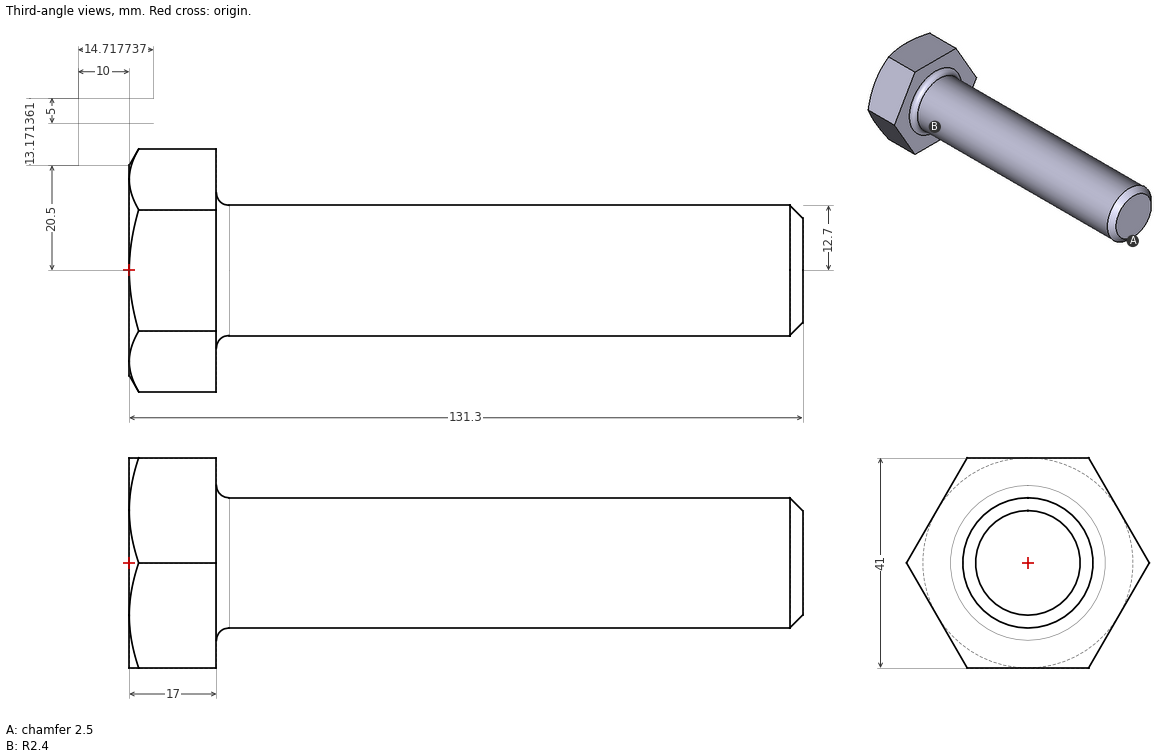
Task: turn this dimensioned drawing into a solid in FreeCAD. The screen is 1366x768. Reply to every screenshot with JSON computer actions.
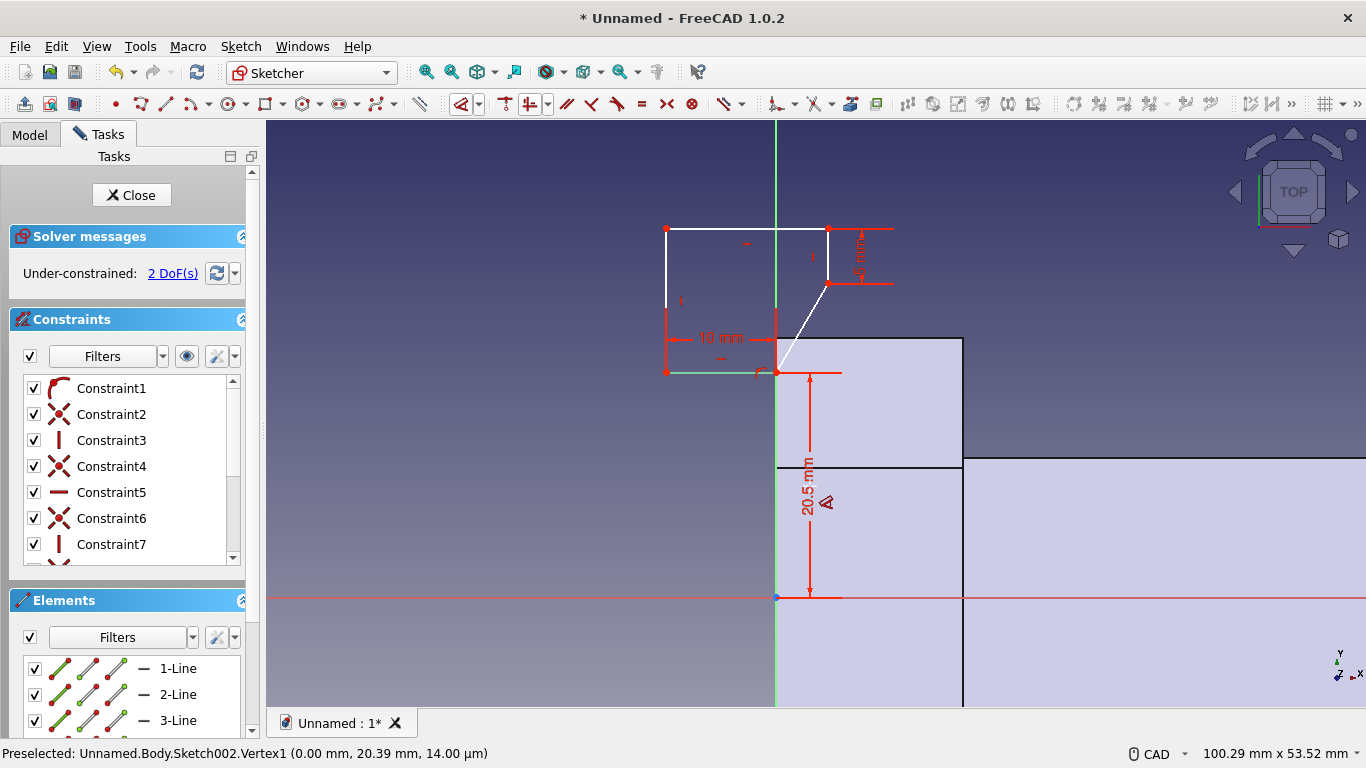
{"action": "left_click", "coordinate": [780, 229]}
{"action": "left_click", "coordinate": [747, 195]}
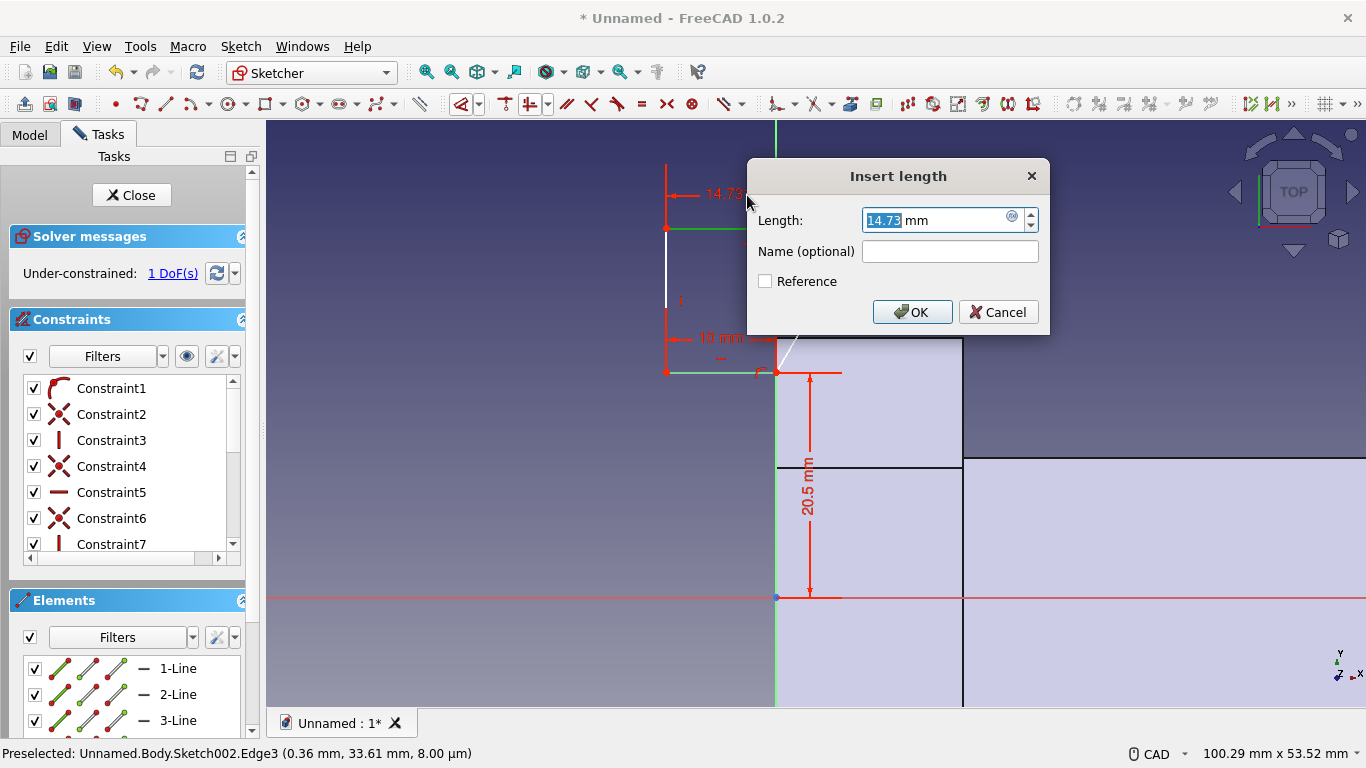
{"action": "type", "text": "14.717737"}
{"action": "key", "text": "Return"}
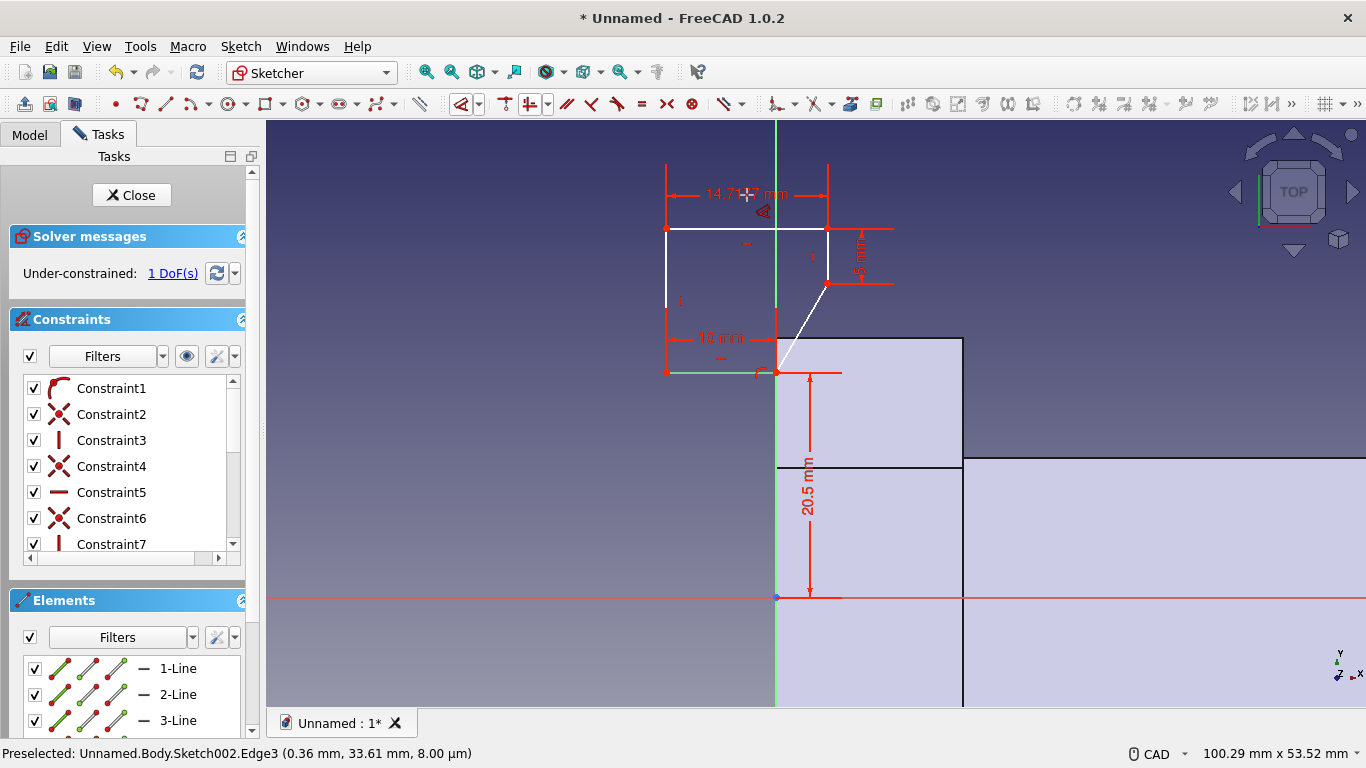
{"action": "left_click", "coordinate": [666, 272]}
{"action": "left_click", "coordinate": [632, 301]}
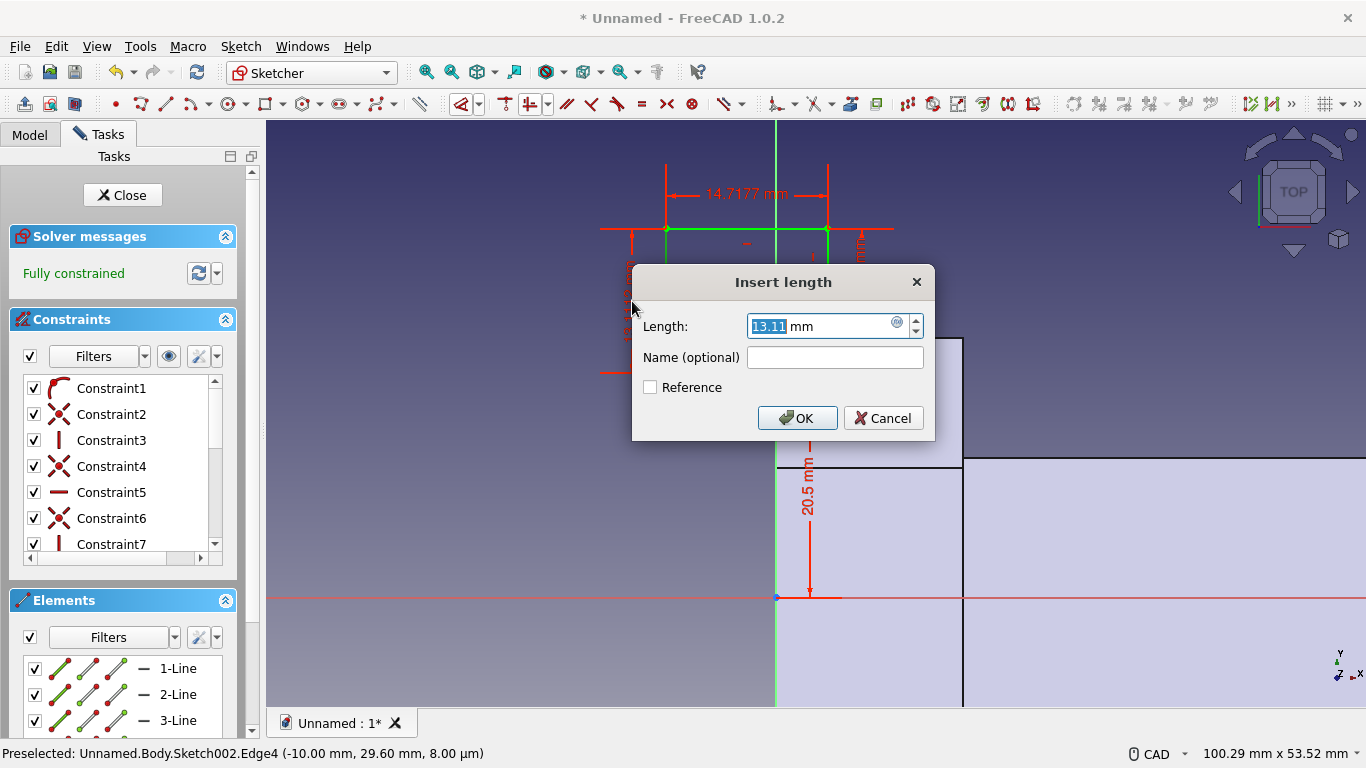
{"action": "type", "text": "13.171361"}
{"action": "key", "text": "Return"}
{"action": "key", "text": "Escape"}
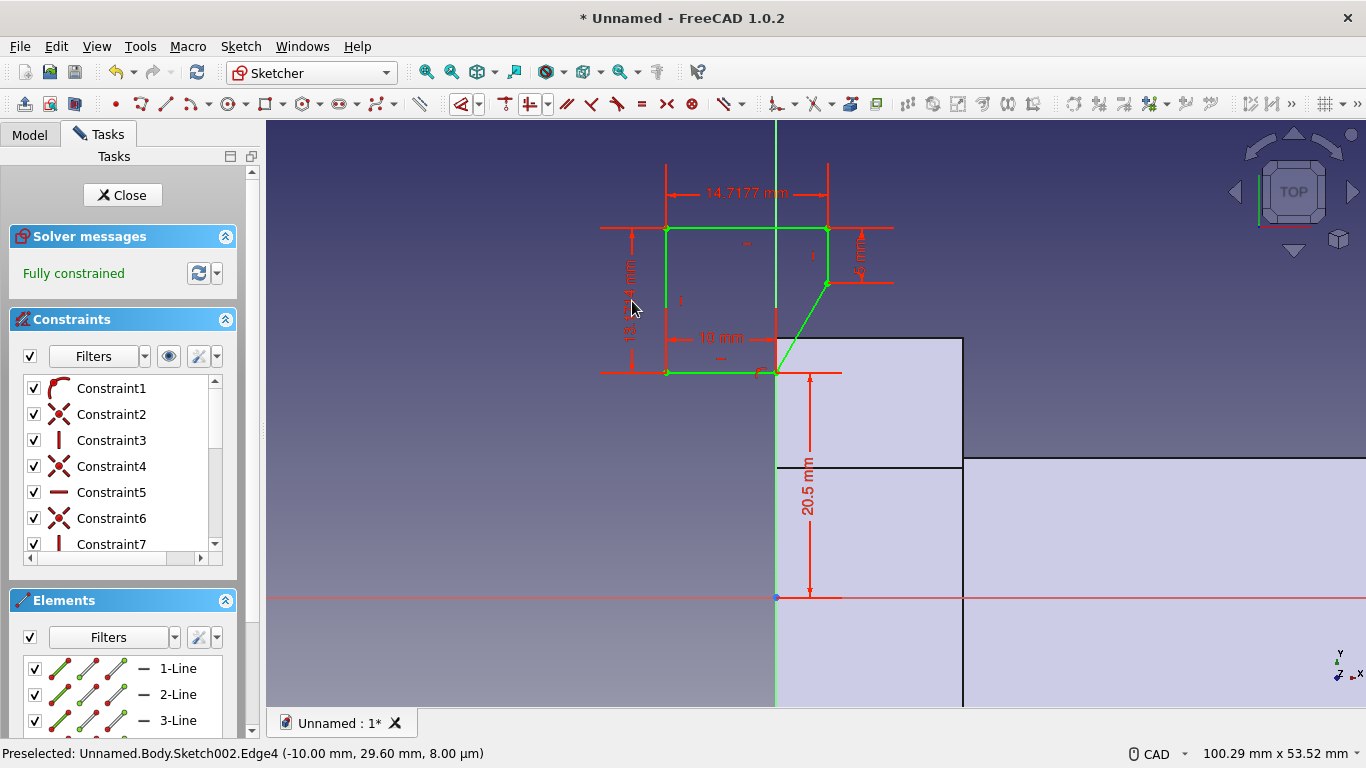
{"action": "left_click", "coordinate": [123, 195]}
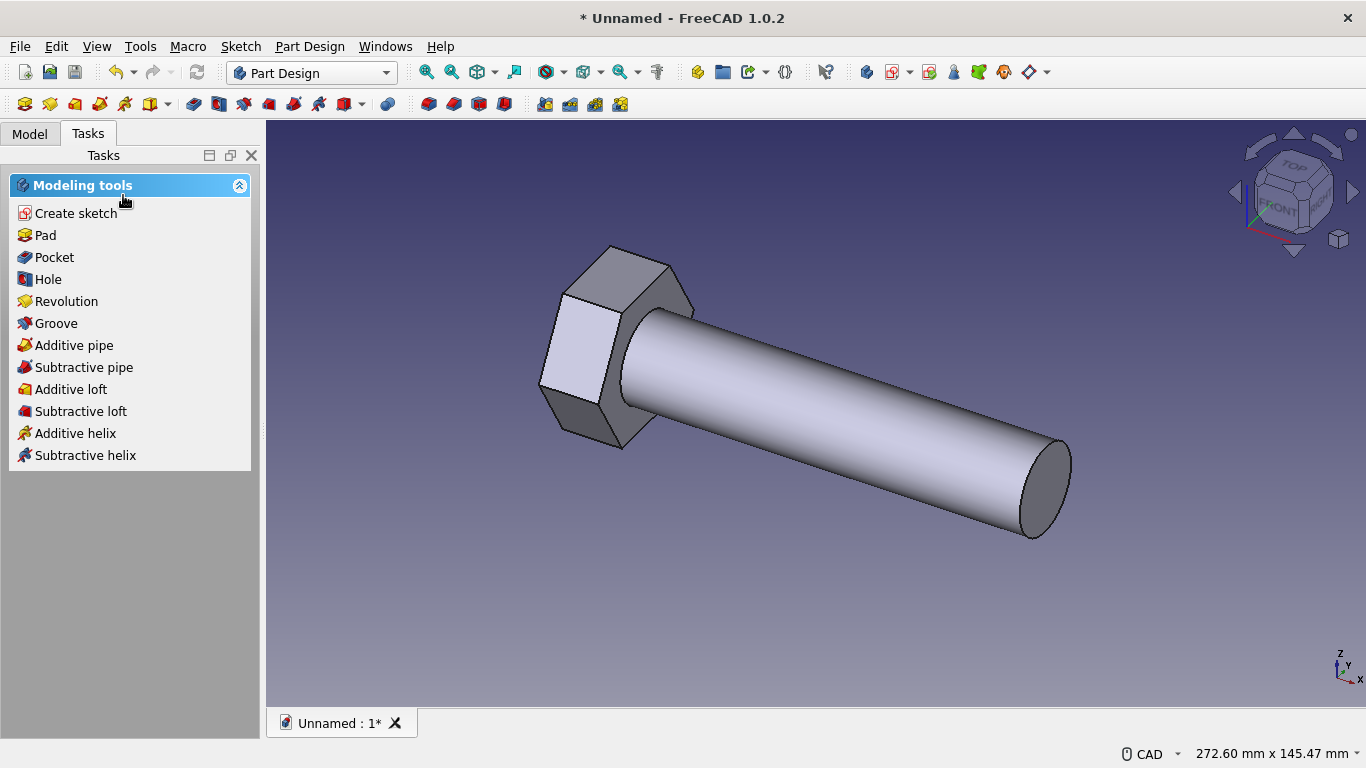
{"action": "left_click", "coordinate": [244, 104]}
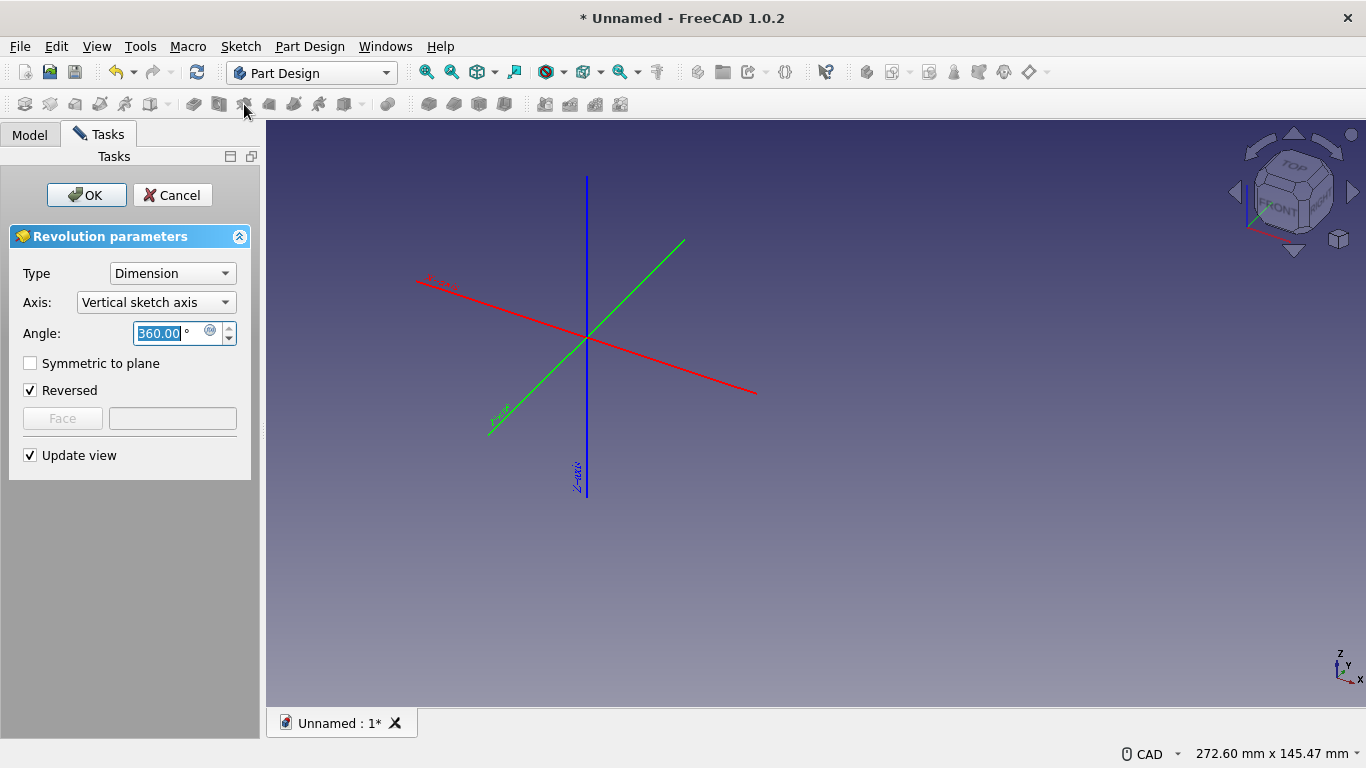
{"action": "left_click", "coordinate": [157, 302]}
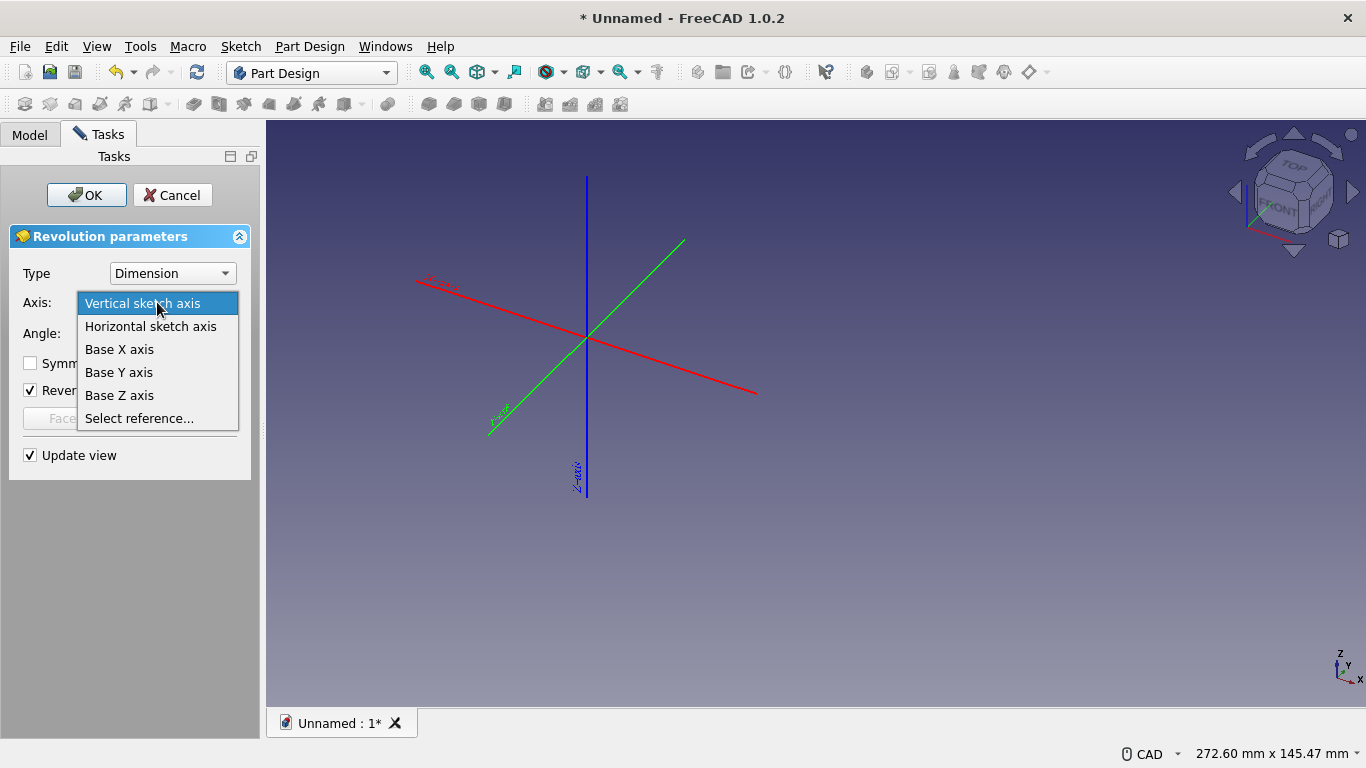
{"action": "left_click", "coordinate": [156, 326]}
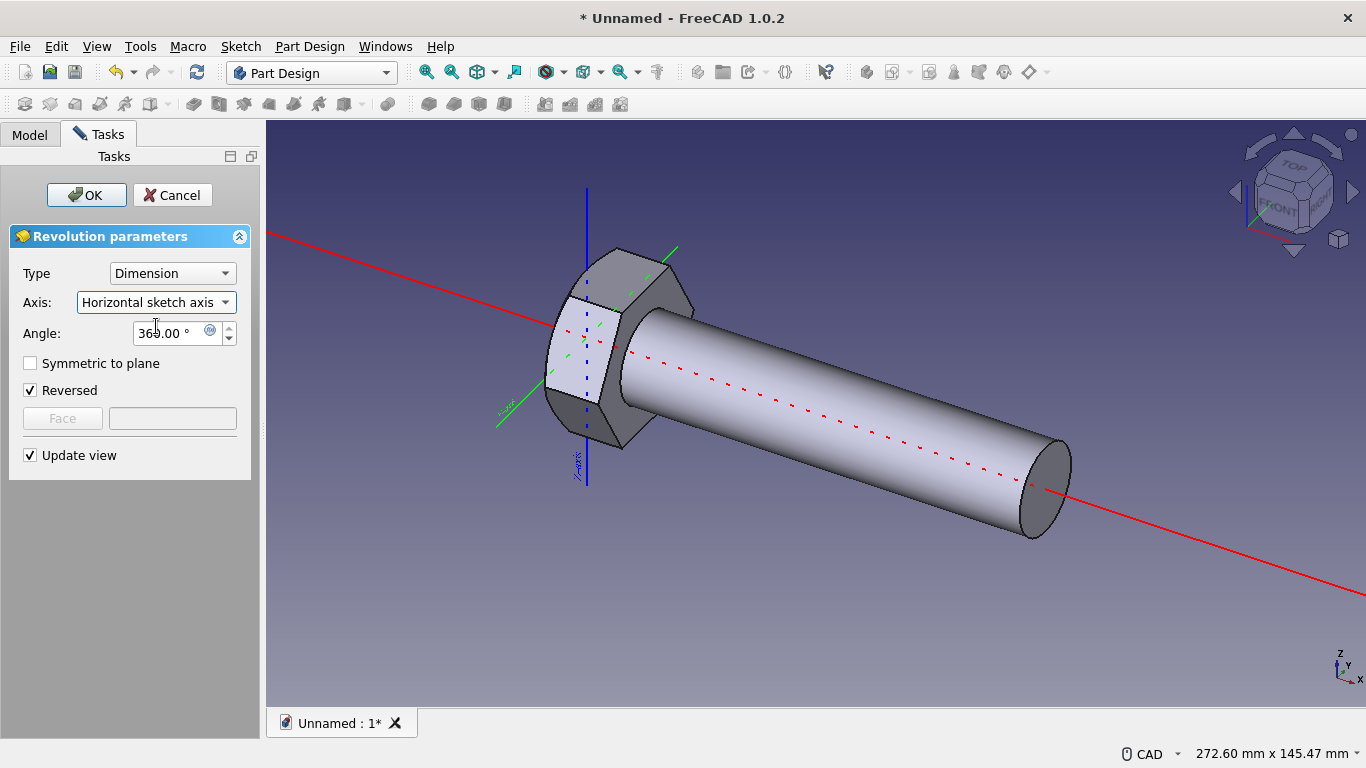
{"action": "left_click", "coordinate": [87, 195]}